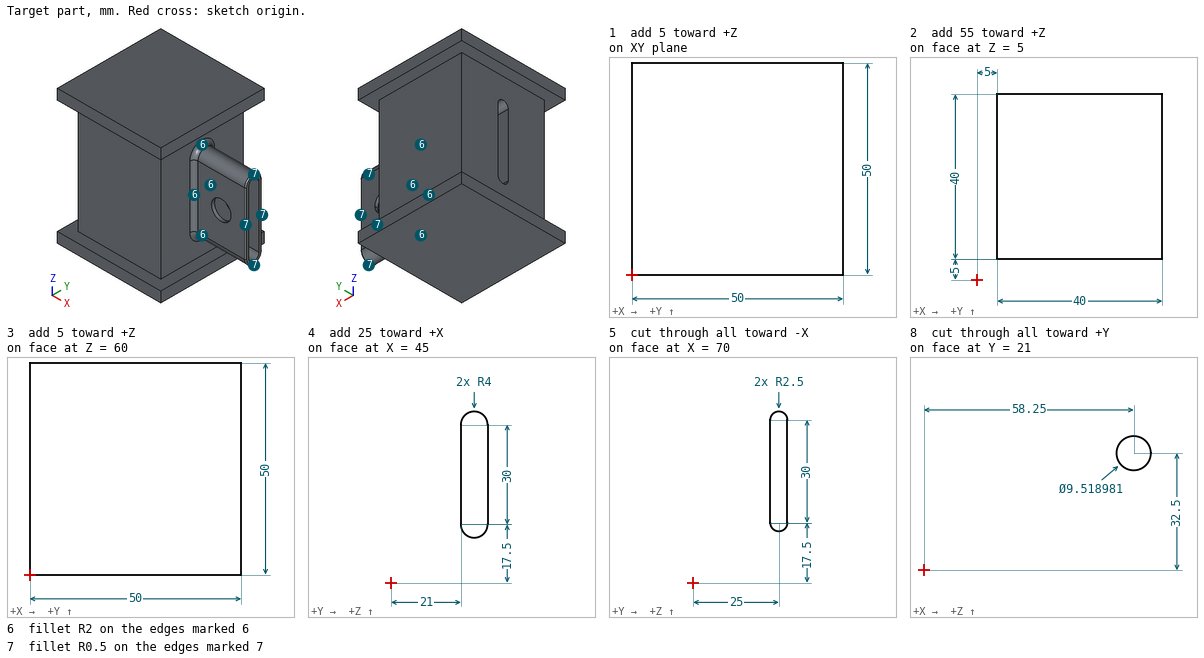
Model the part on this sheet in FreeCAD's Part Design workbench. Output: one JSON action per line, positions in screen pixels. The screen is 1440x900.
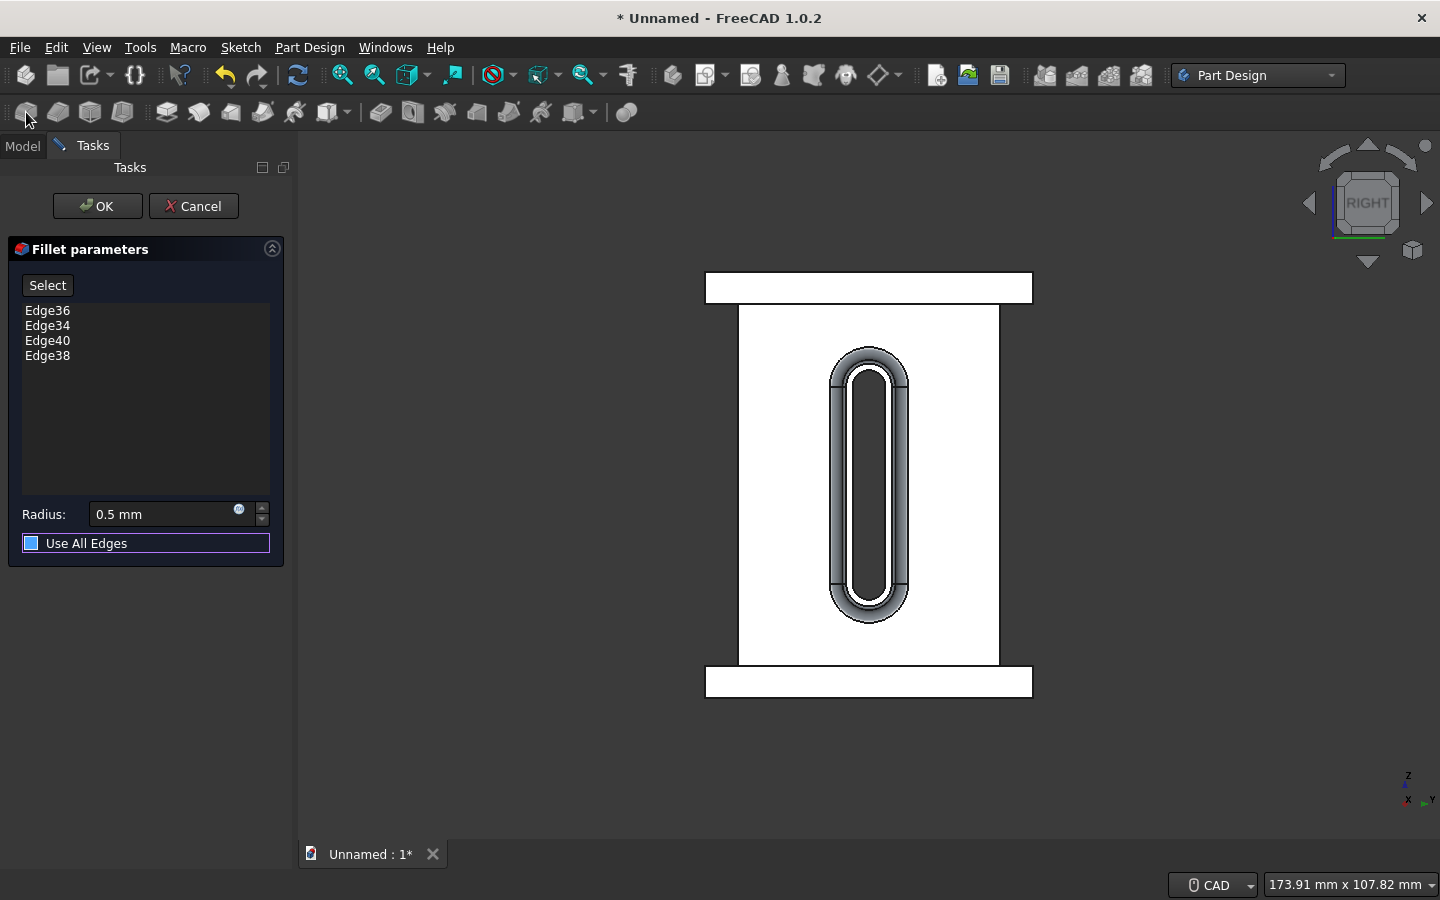
{"action": "left_click", "coordinate": [98, 206]}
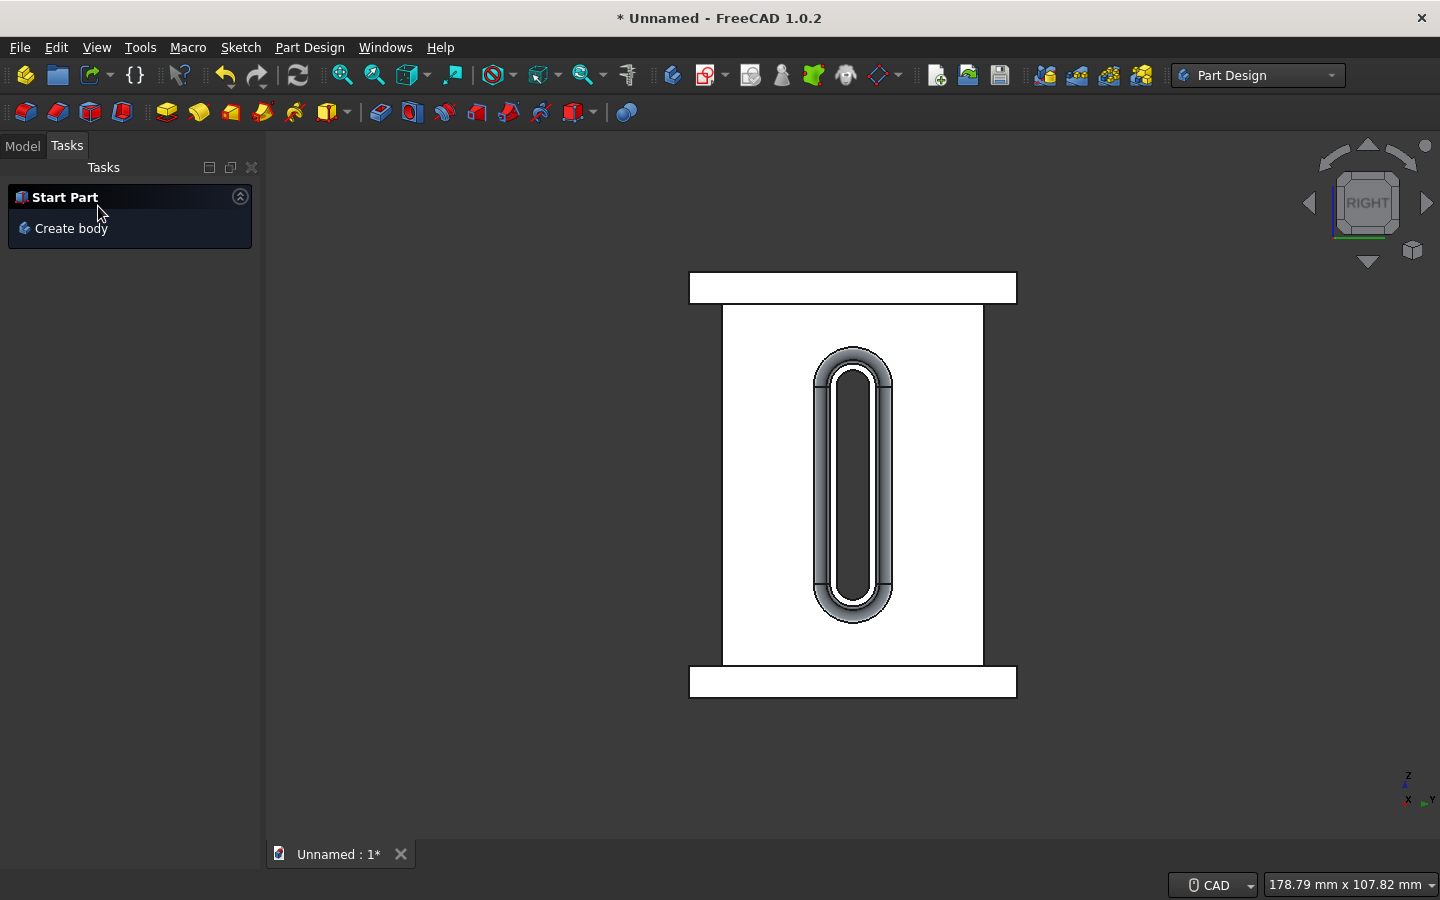
{"action": "key", "text": "0"}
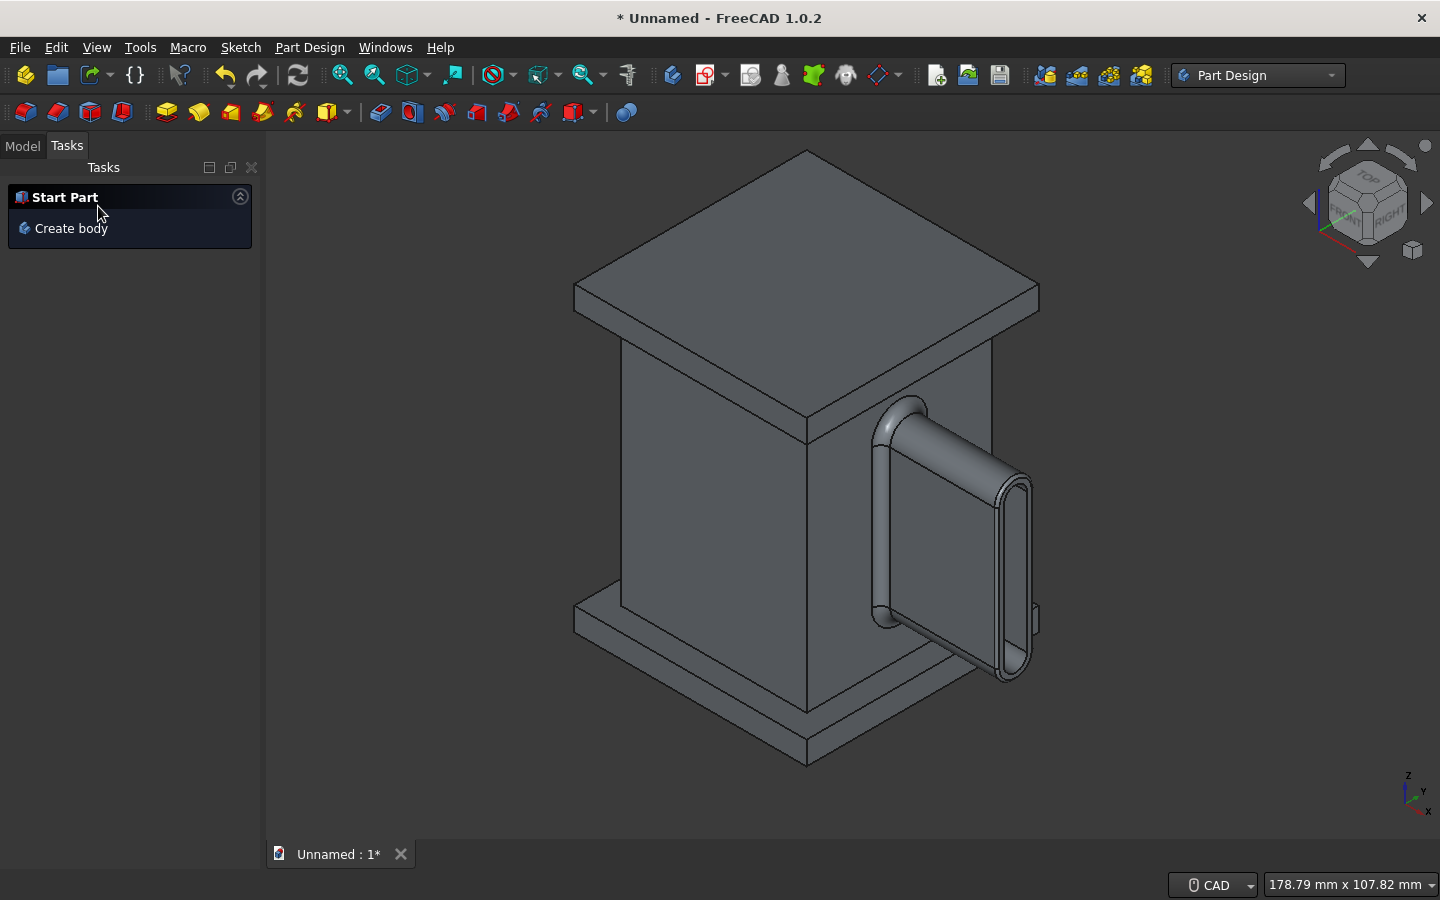
{"action": "left_click", "coordinate": [942, 557]}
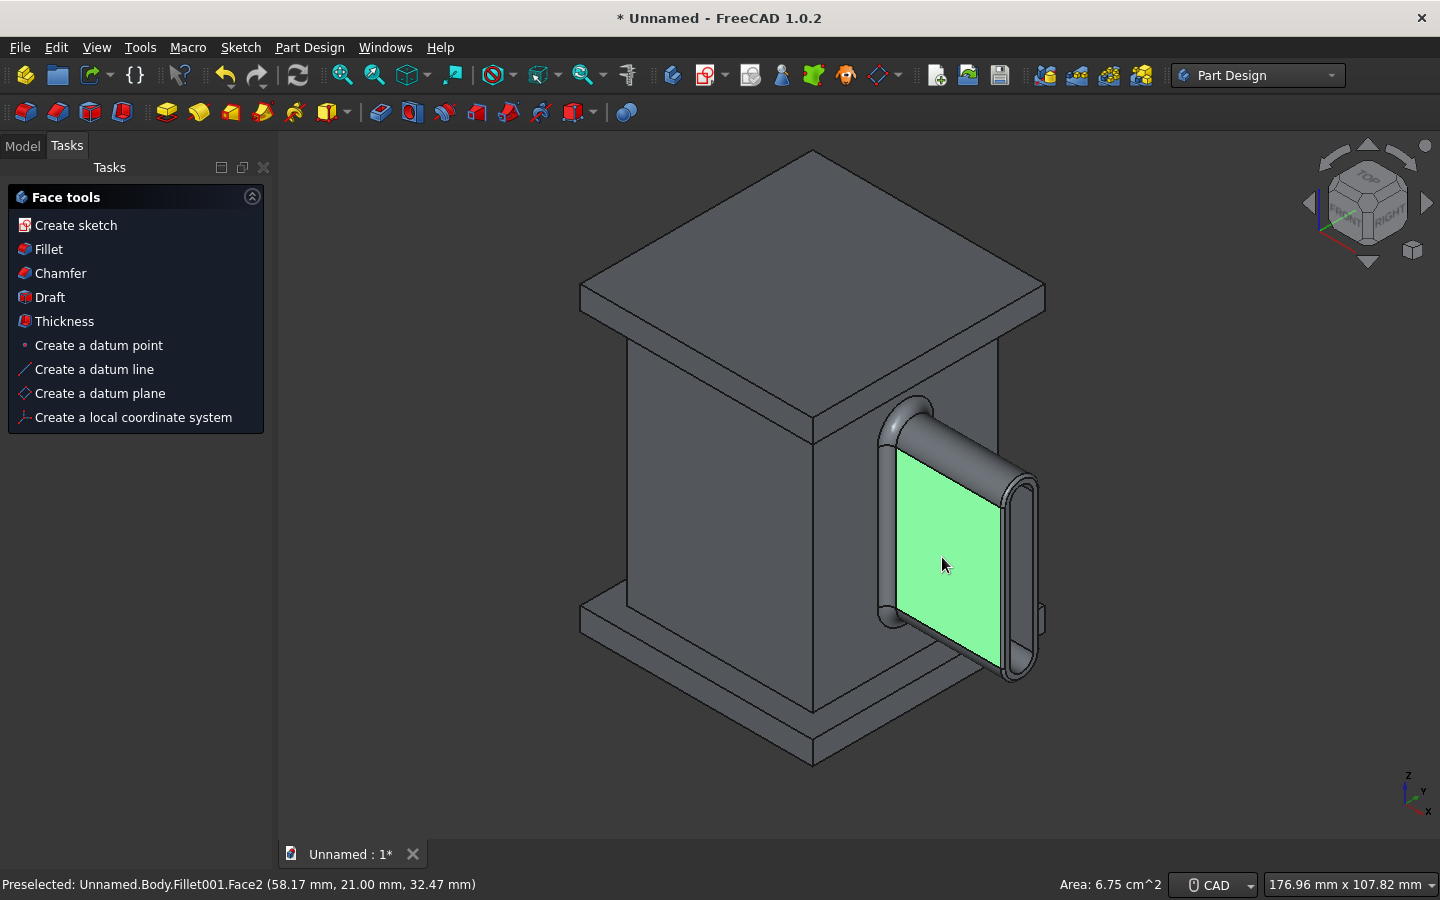
{"action": "left_click", "coordinate": [706, 76]}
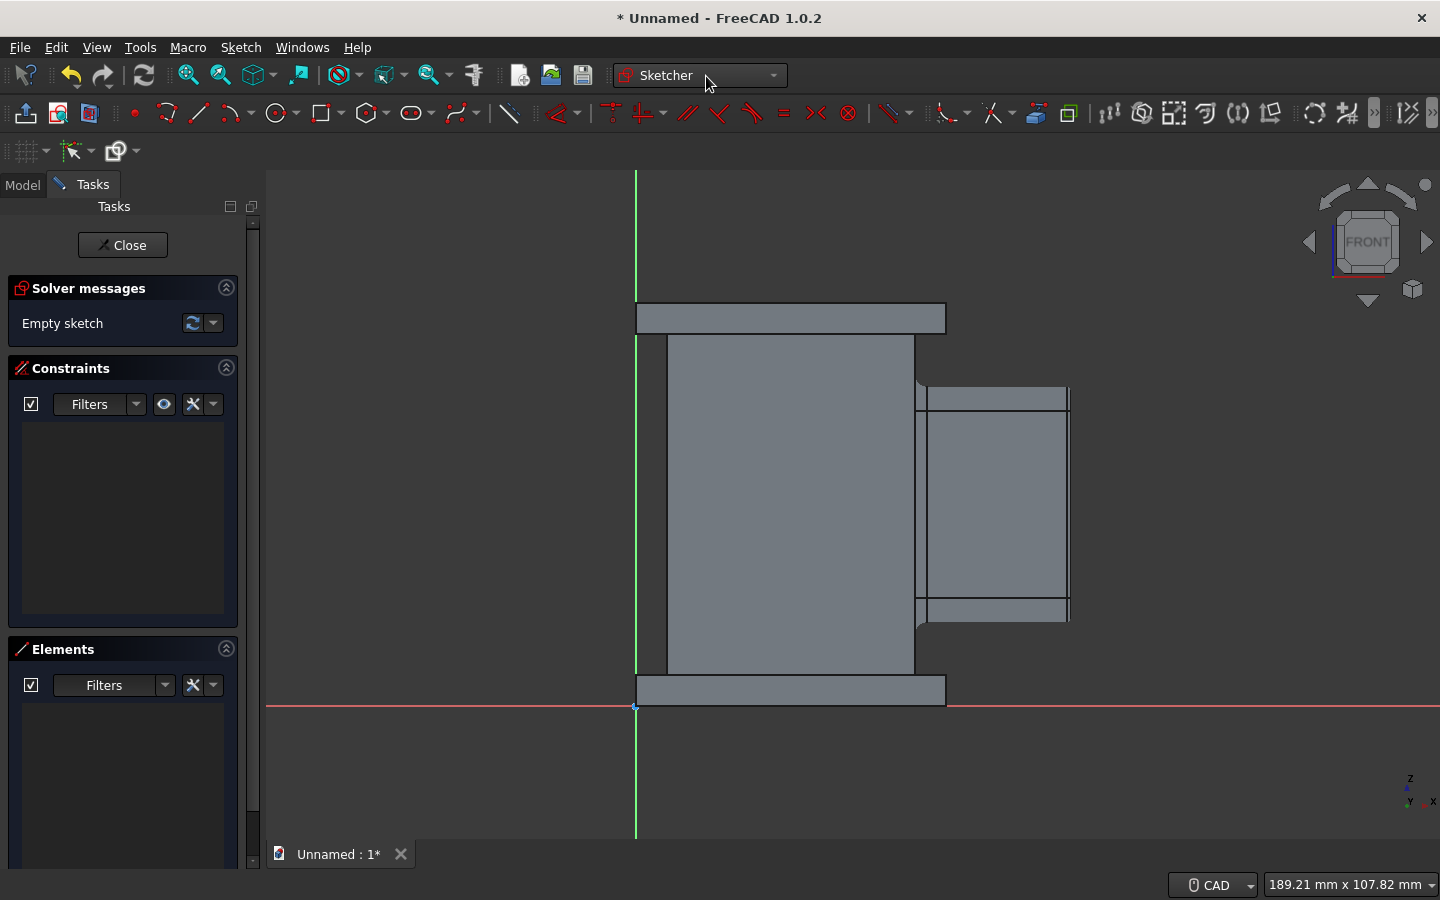
{"action": "left_click", "coordinate": [90, 114]}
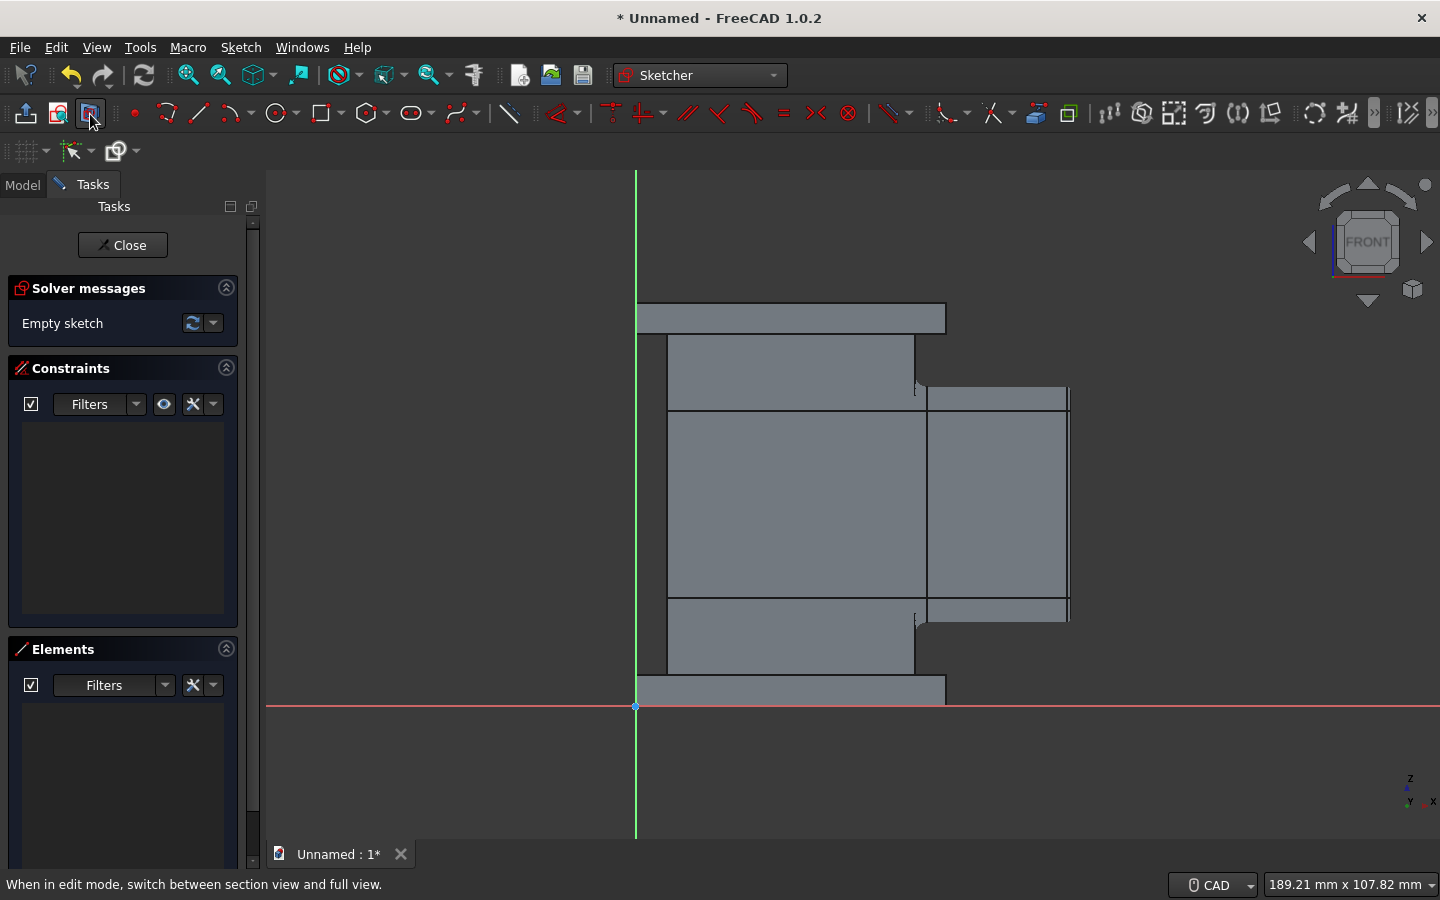
{"action": "scroll", "coordinate": [1031, 504], "scroll_direction": "up", "scroll_amount": 10}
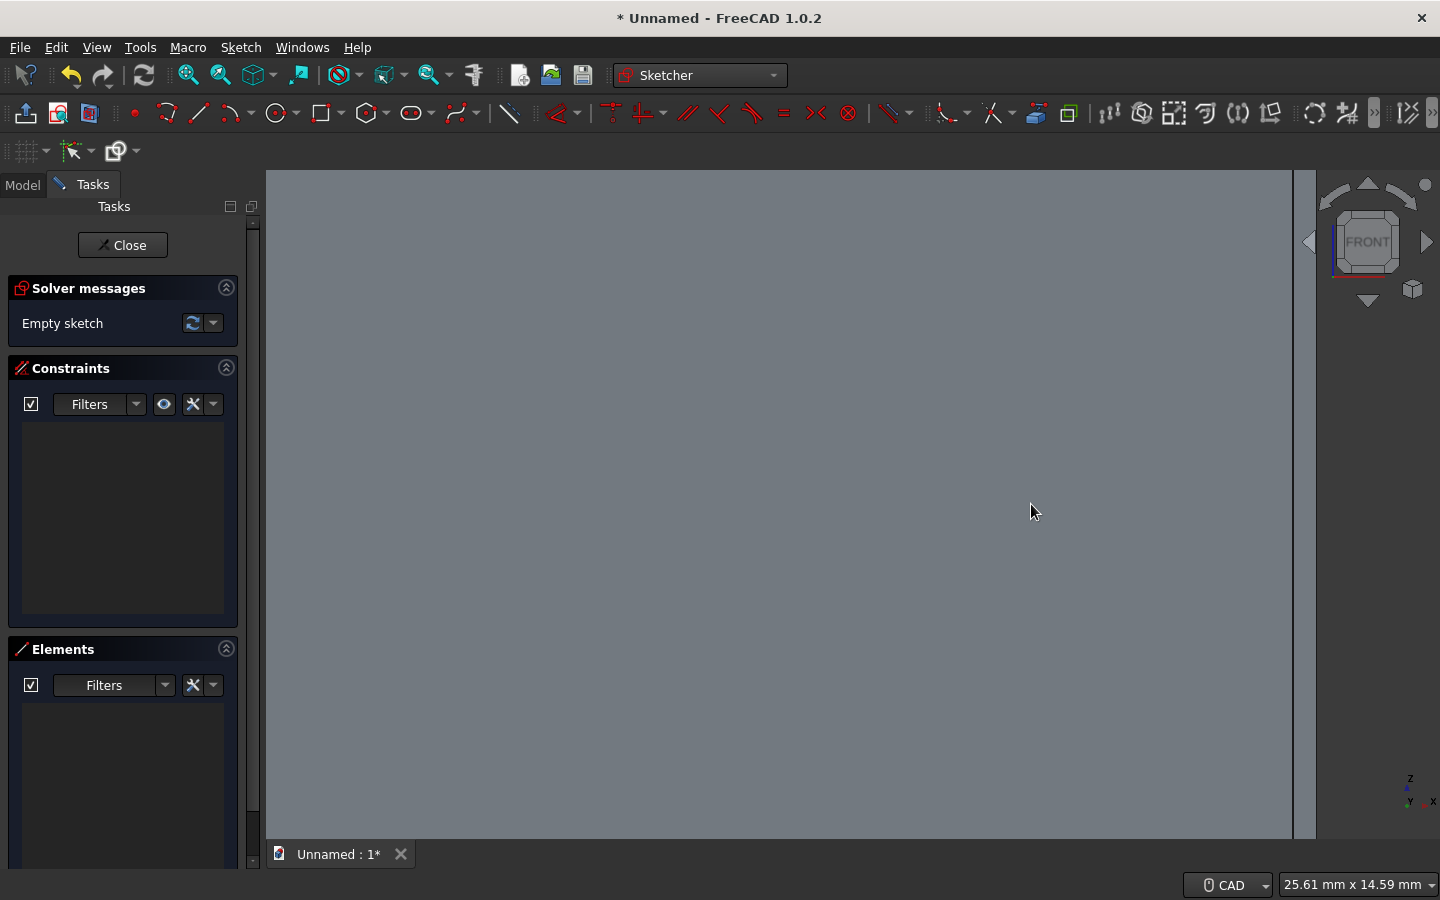
{"action": "left_click", "coordinate": [276, 114]}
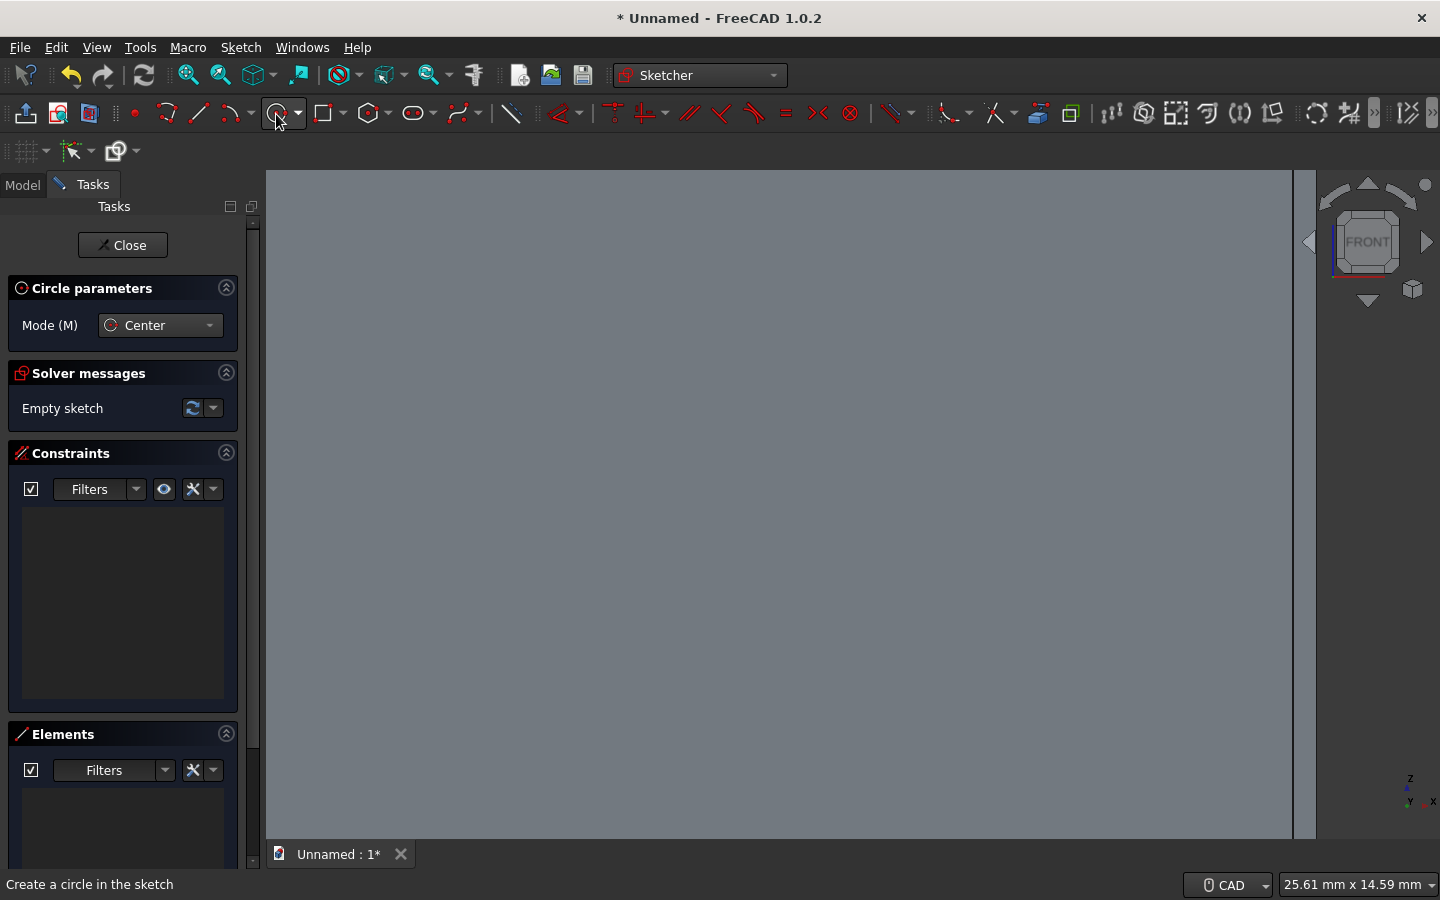
{"action": "left_click", "coordinate": [778, 504]}
{"action": "left_click", "coordinate": [932, 350]}
{"action": "key", "text": "Escape"}